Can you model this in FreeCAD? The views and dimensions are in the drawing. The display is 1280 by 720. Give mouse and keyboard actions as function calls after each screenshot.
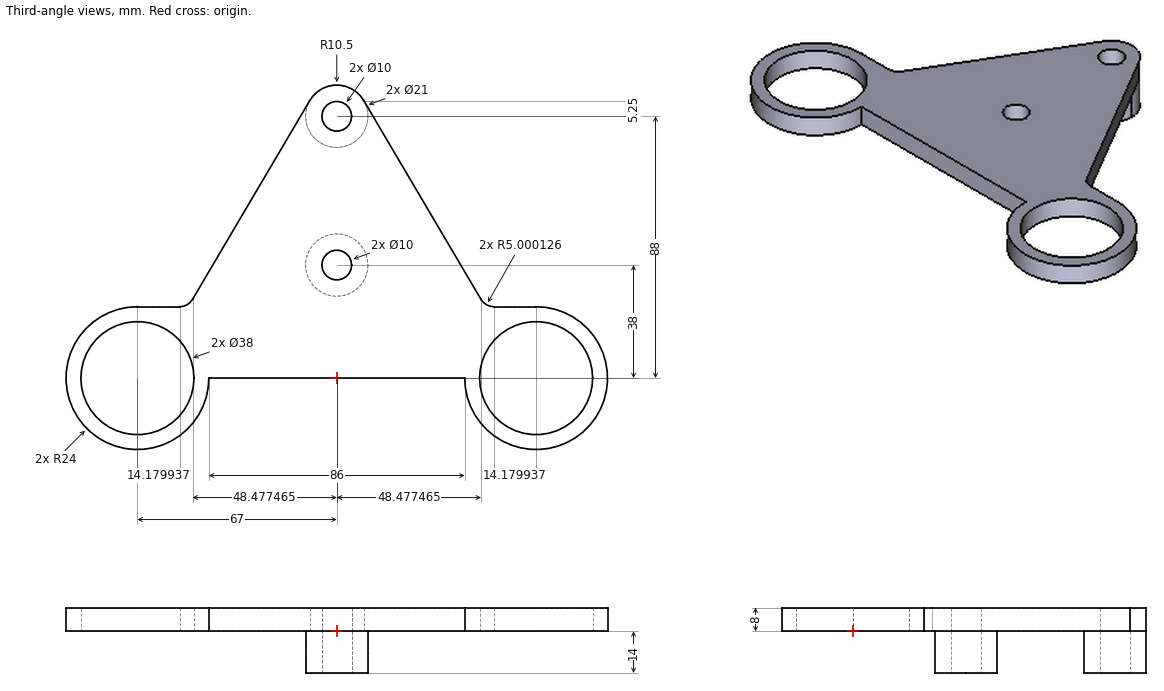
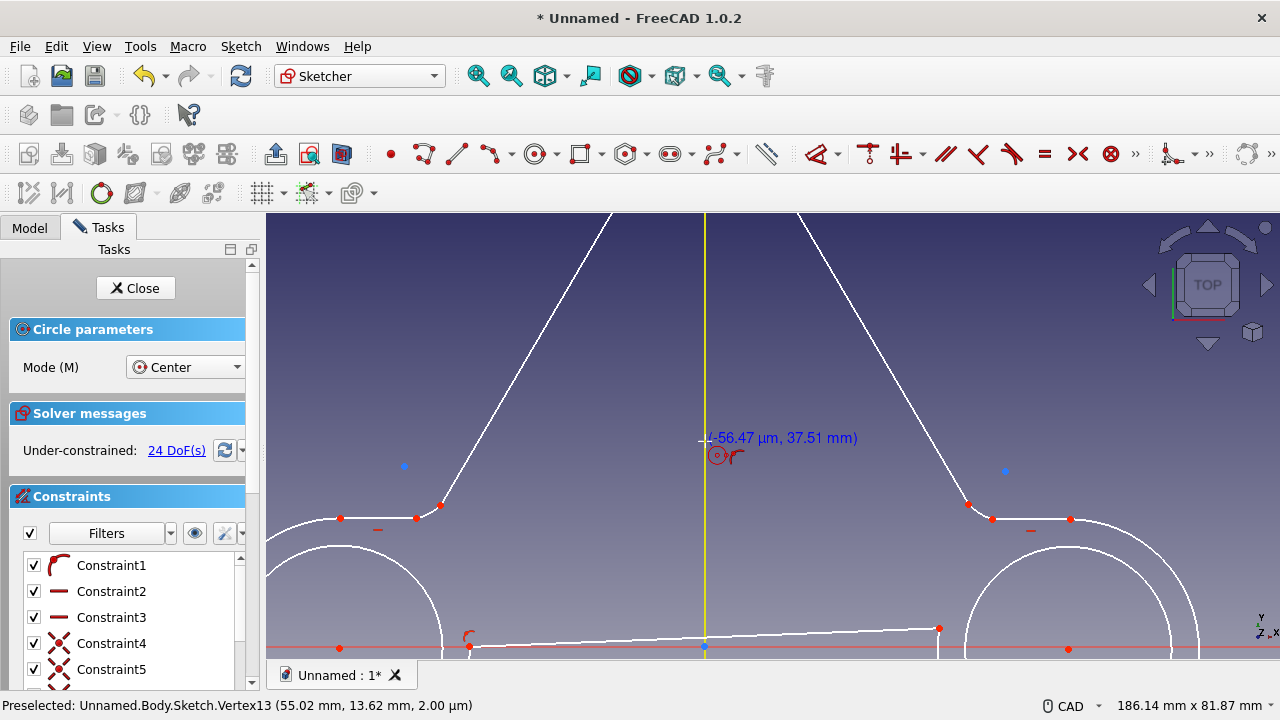
click(705, 440)
click(724, 421)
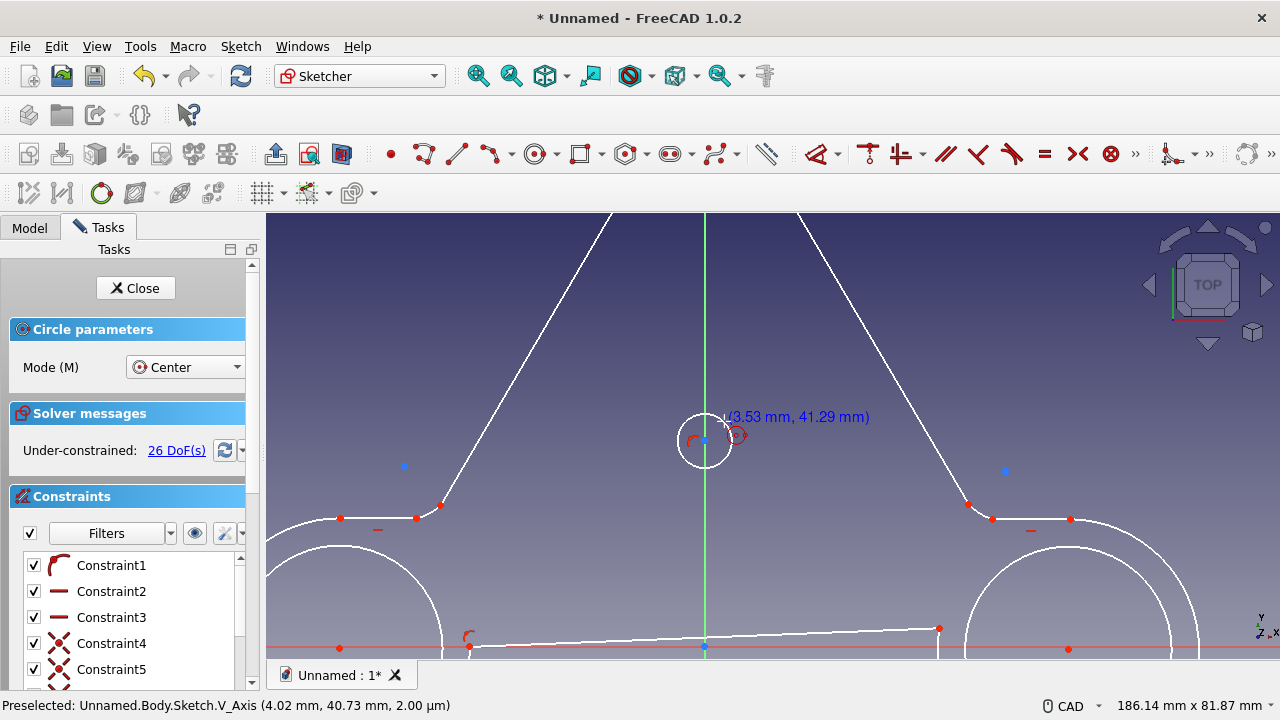
scroll(704, 441, down, 4)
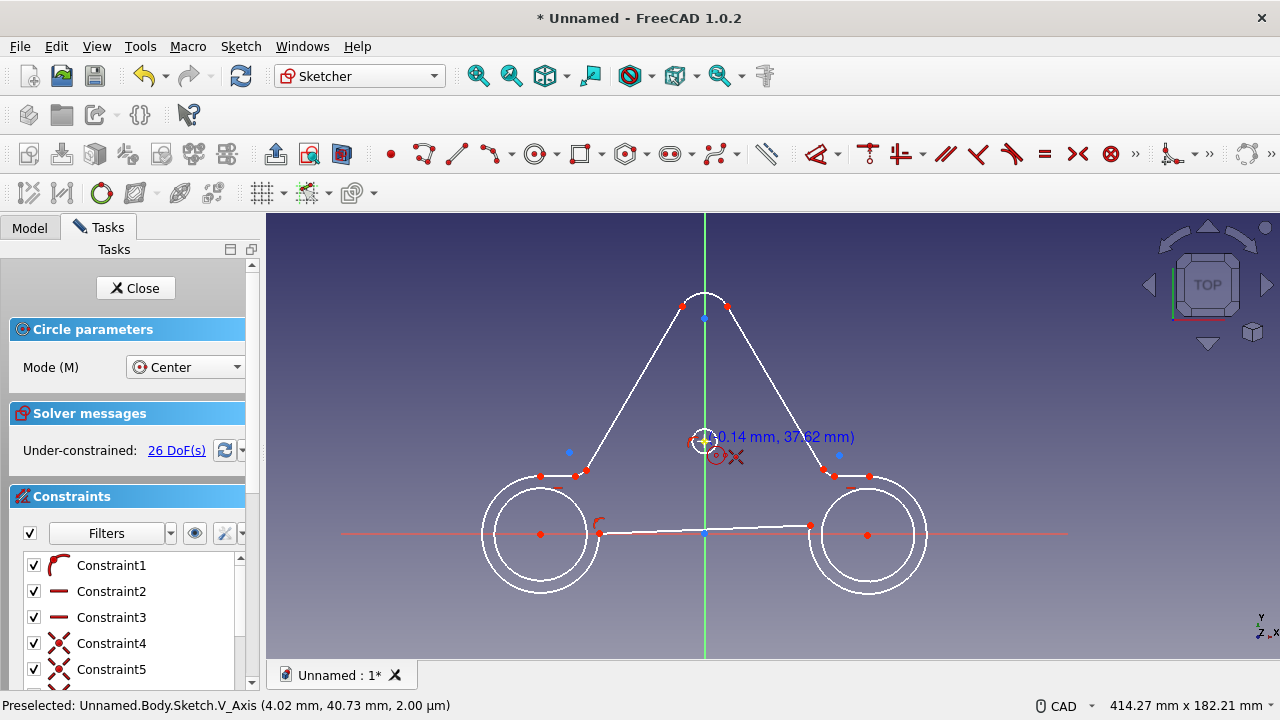
scroll(705, 318, up, 4)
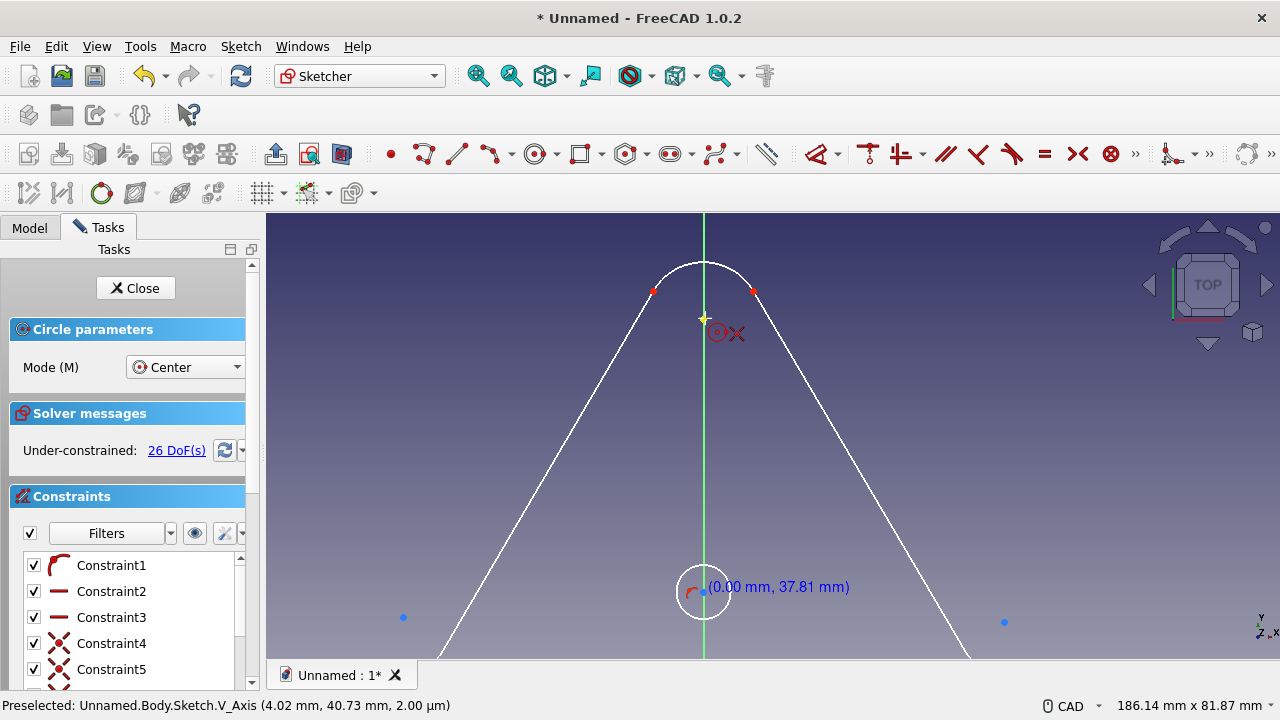
click(704, 319)
click(723, 299)
key(Escape)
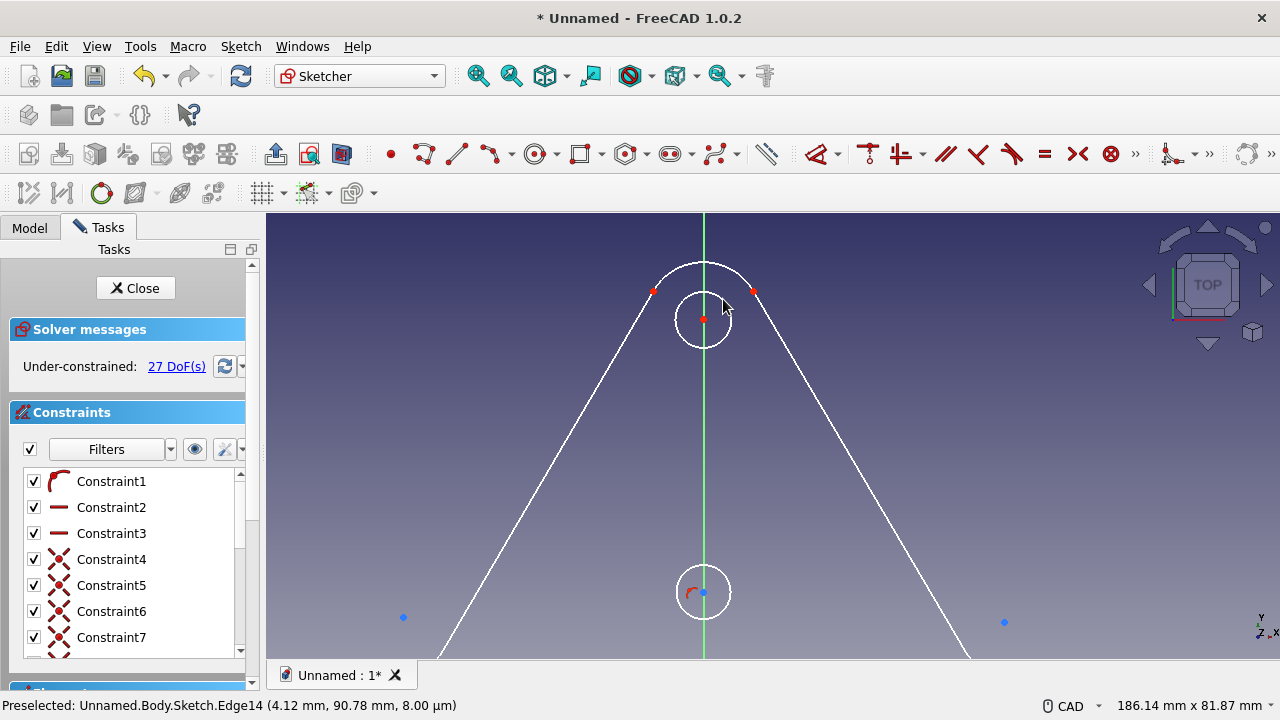
scroll(705, 317, down, 4)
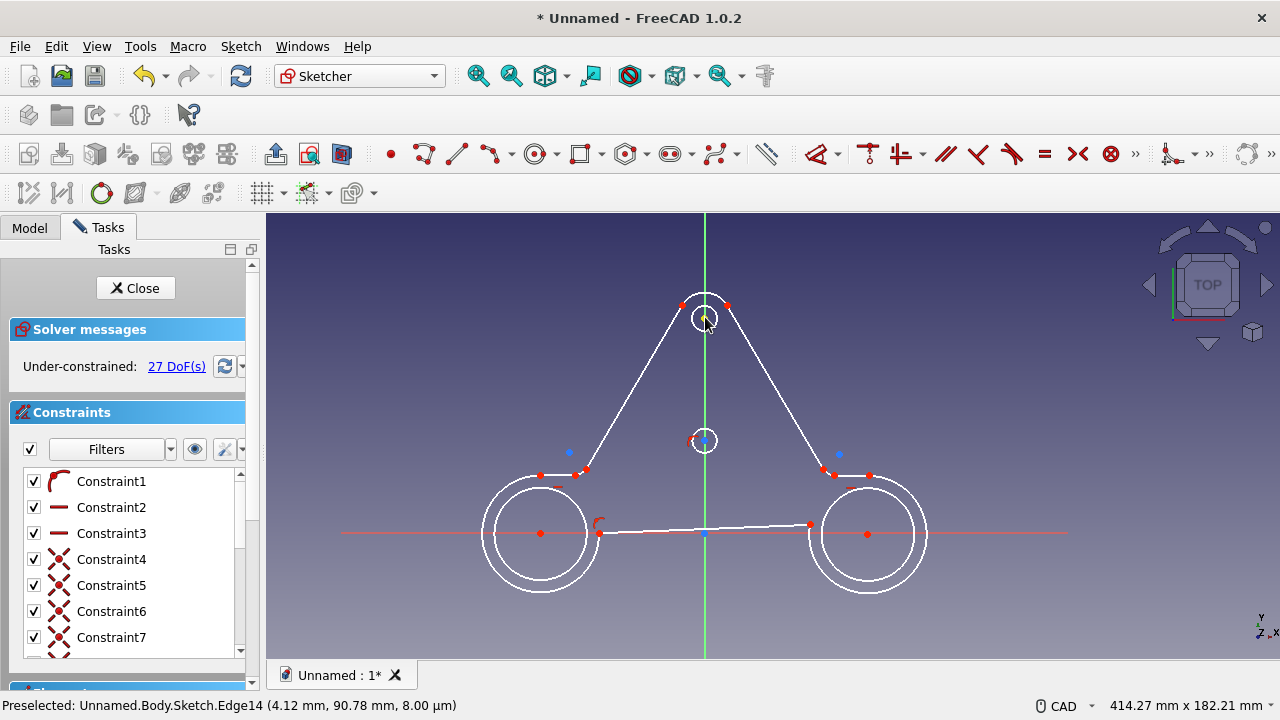
scroll(859, 476, up, 2)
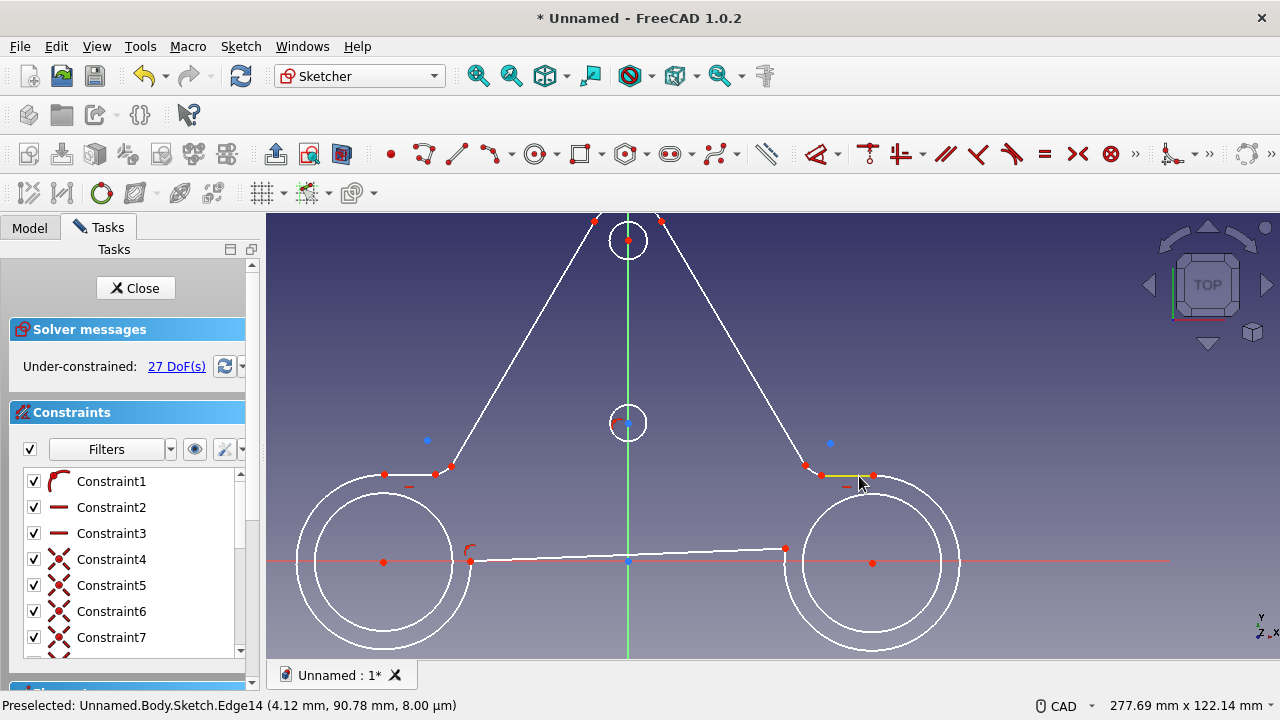
click(858, 476)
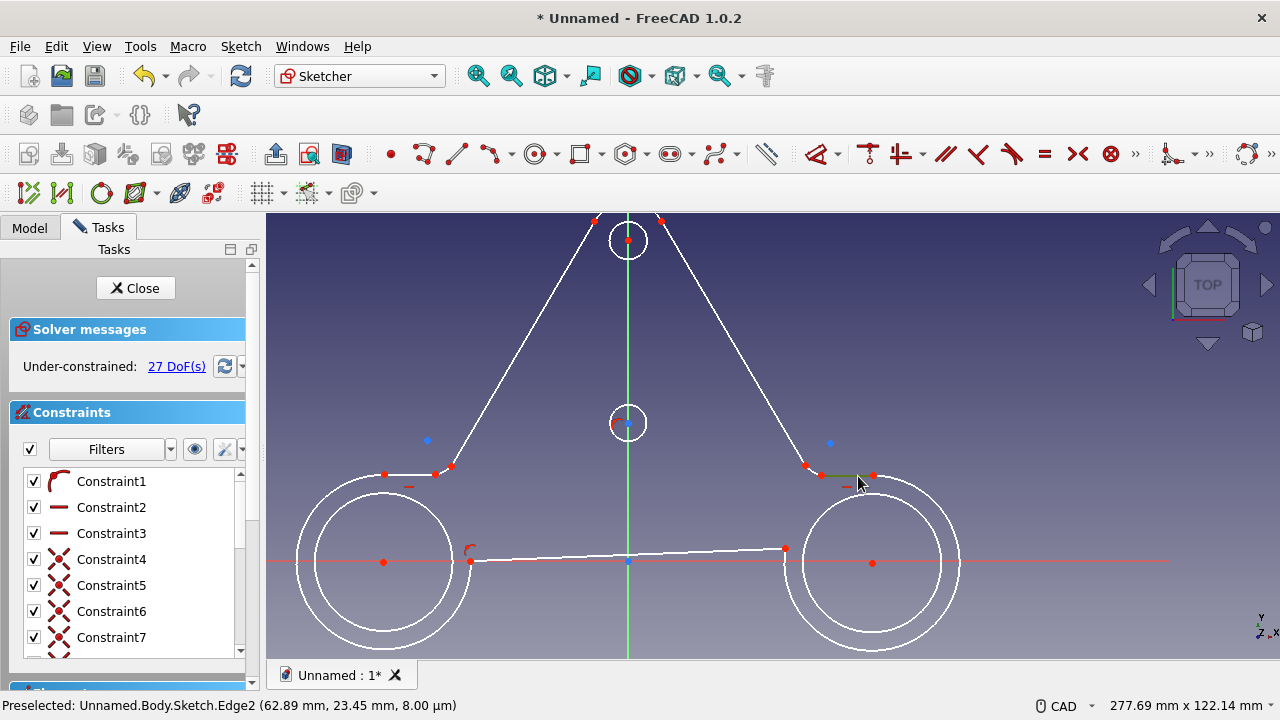
click(928, 631)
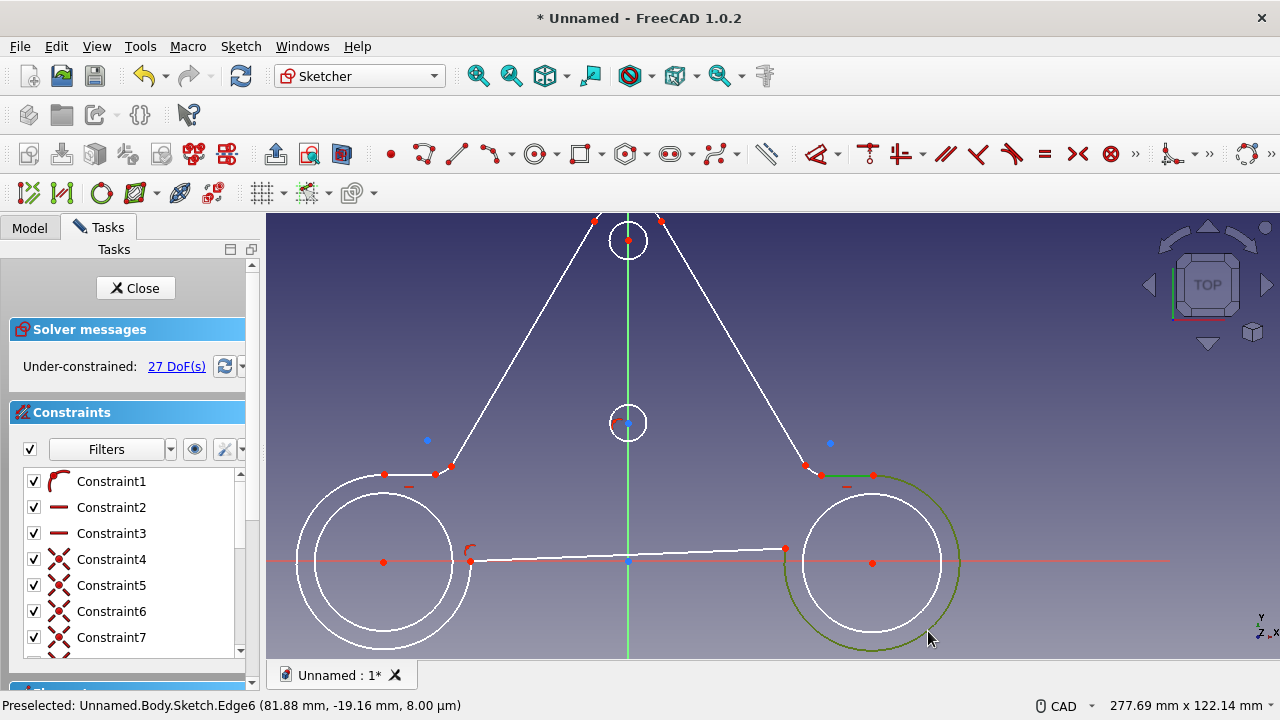
click(1012, 154)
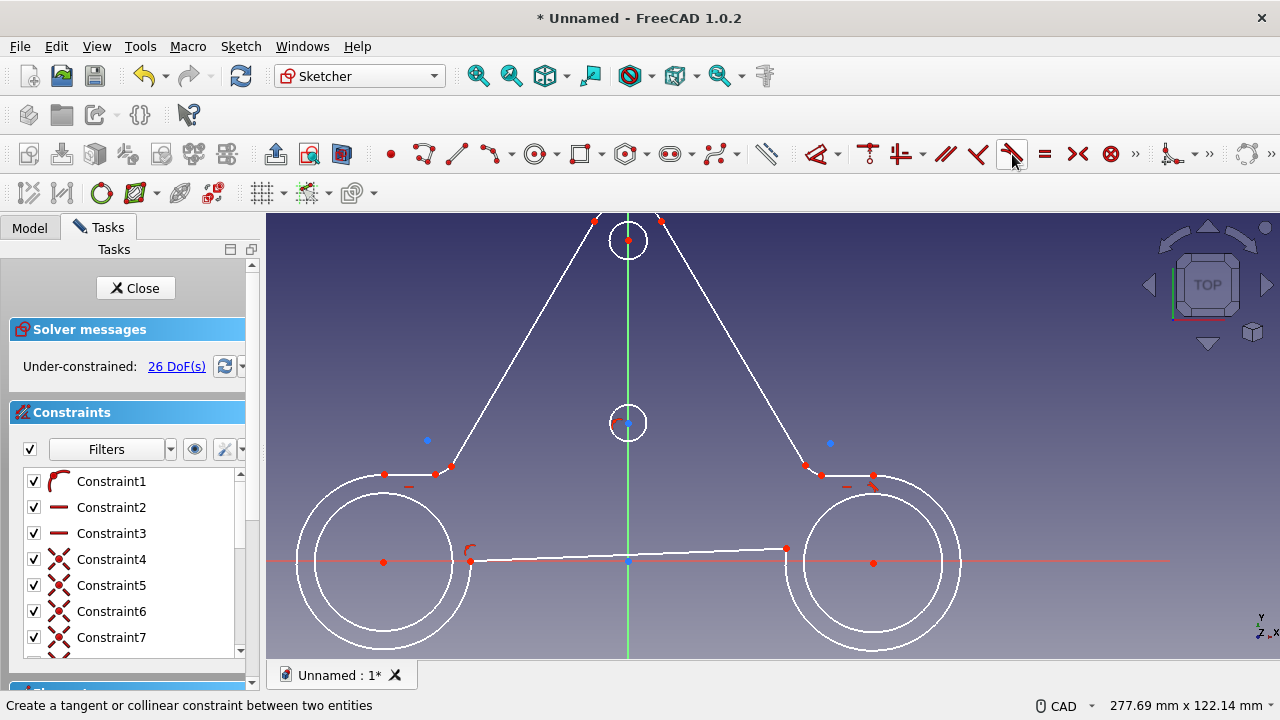
click(762, 392)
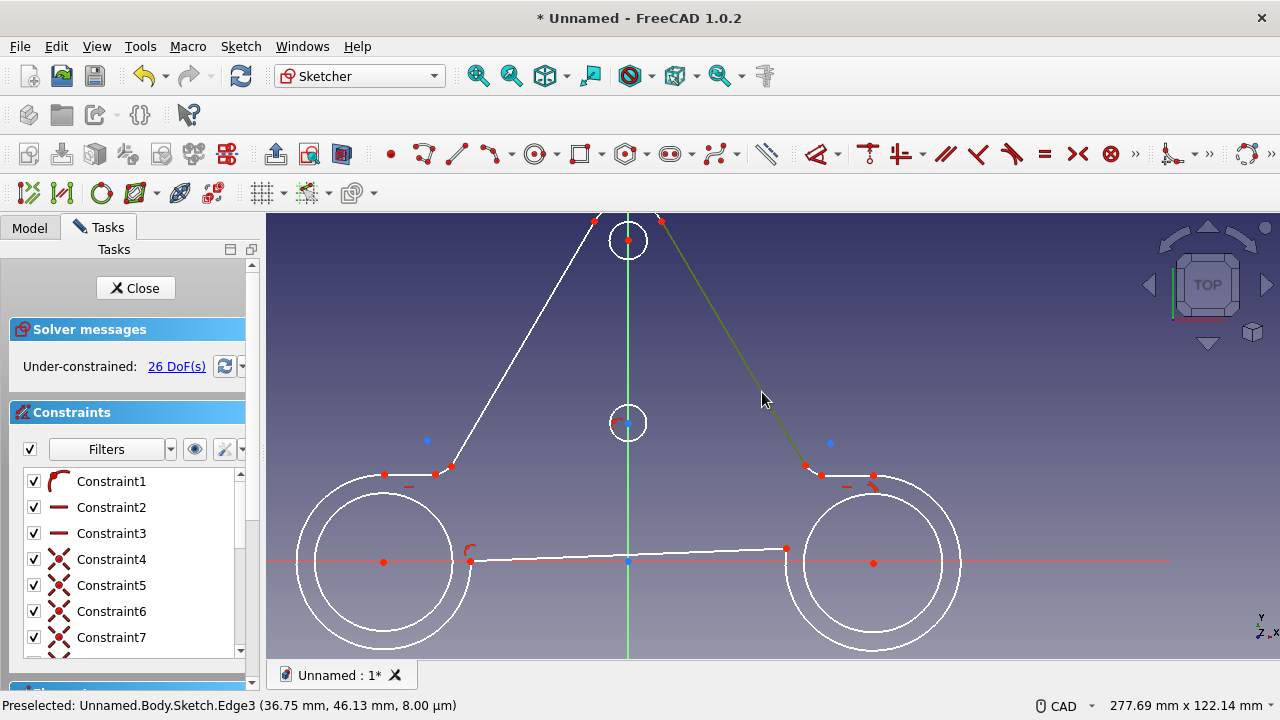
scroll(813, 472, up, 2)